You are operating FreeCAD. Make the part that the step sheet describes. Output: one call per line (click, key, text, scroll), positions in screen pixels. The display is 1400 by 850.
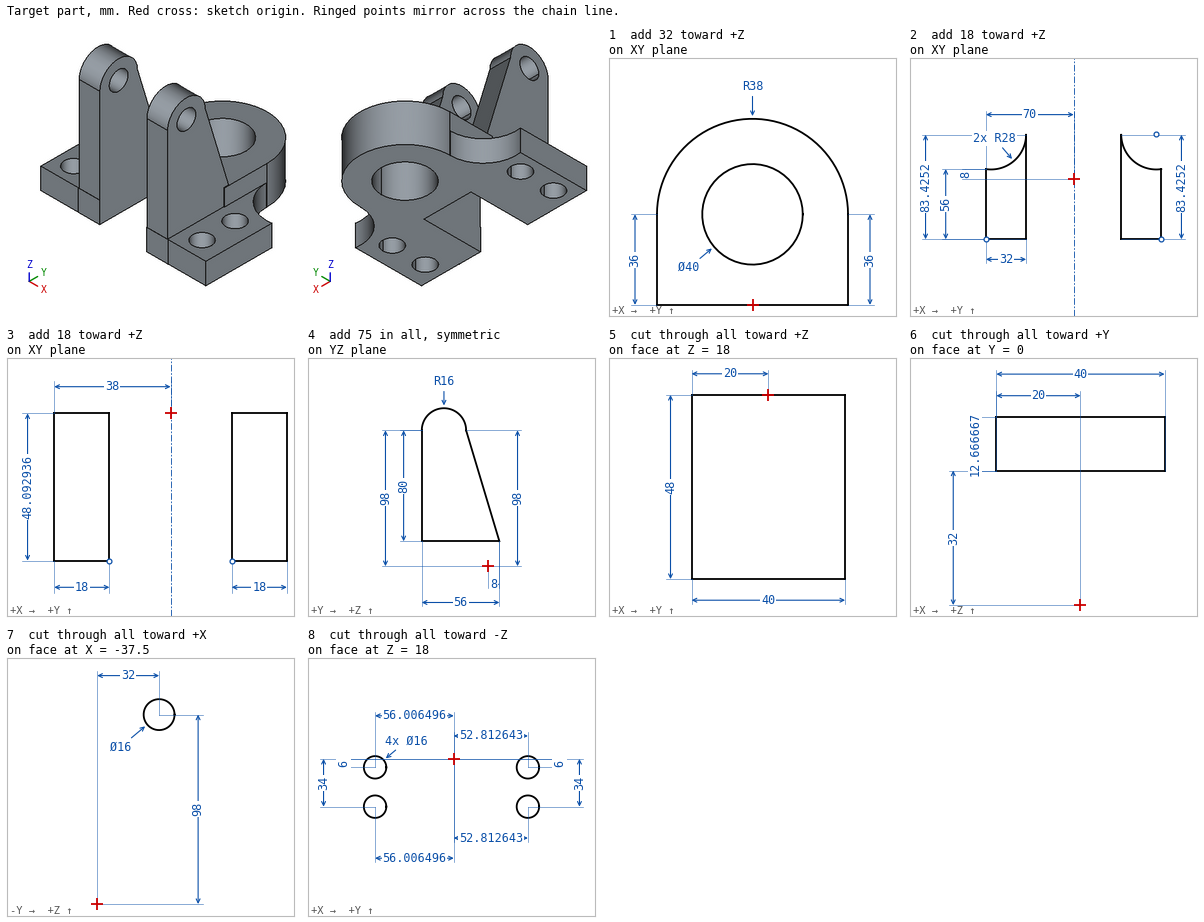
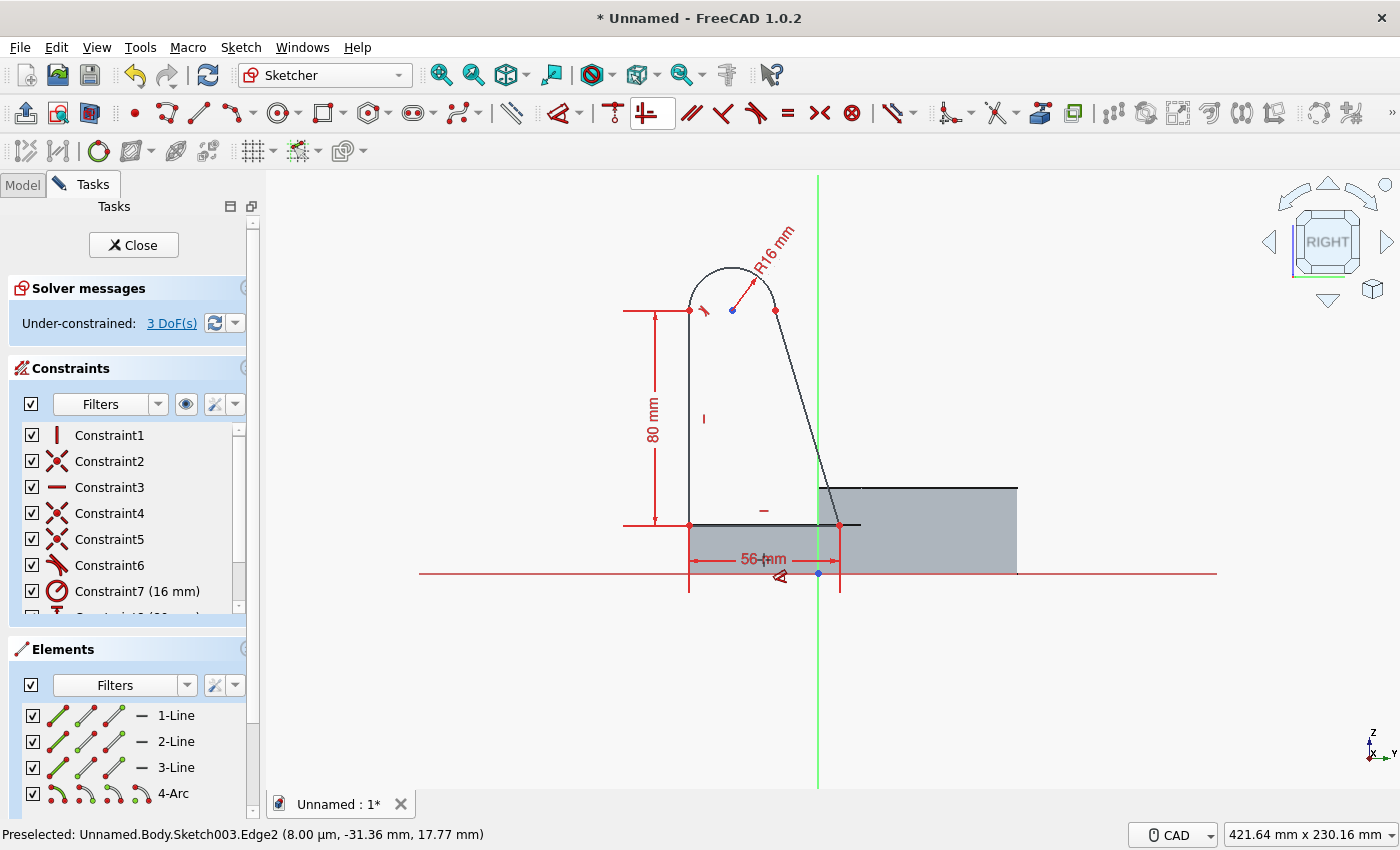
scroll(840, 526, up, 4)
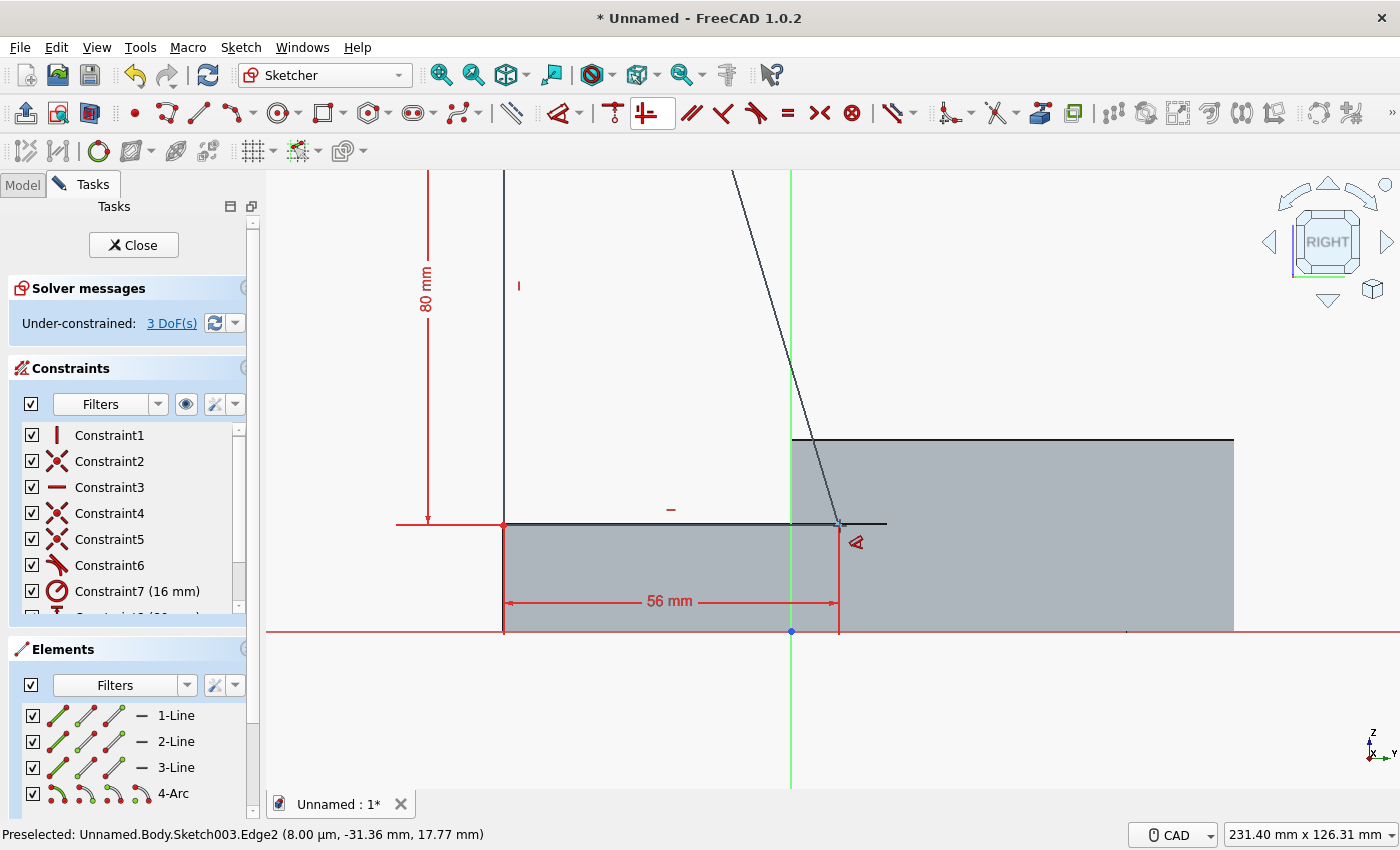
click(839, 525)
click(815, 666)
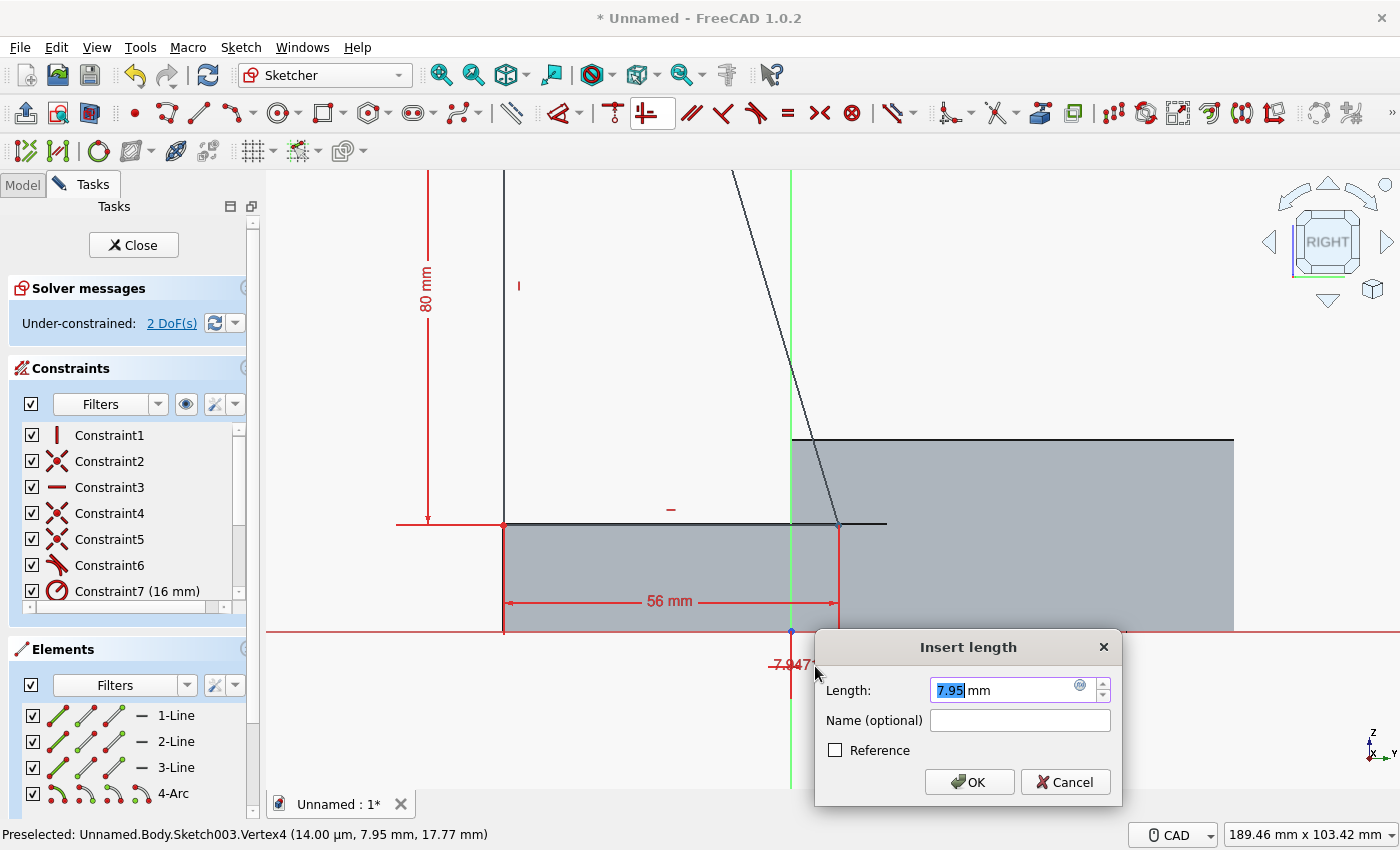
text(8)
key(Return)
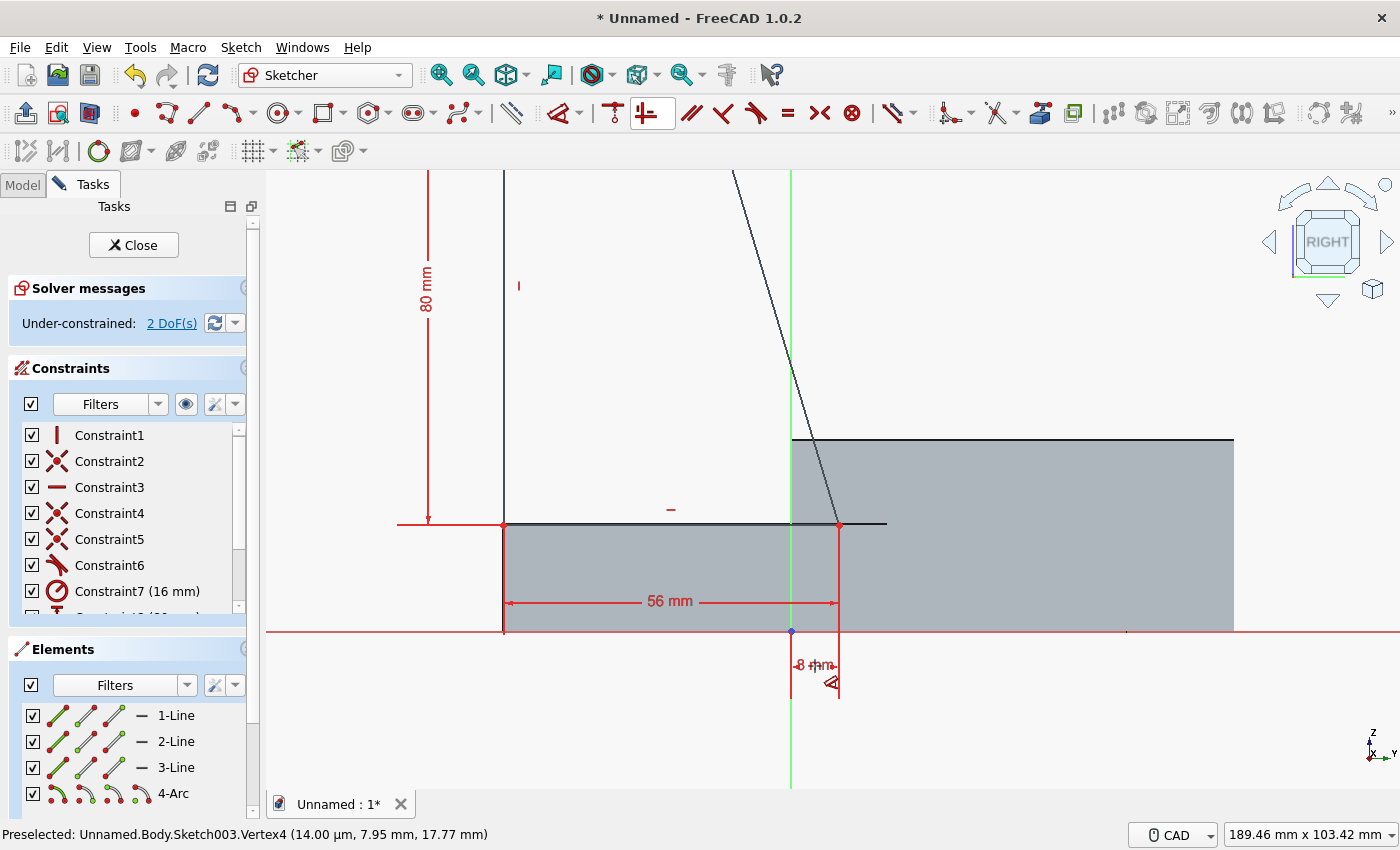
scroll(878, 709, down, 3)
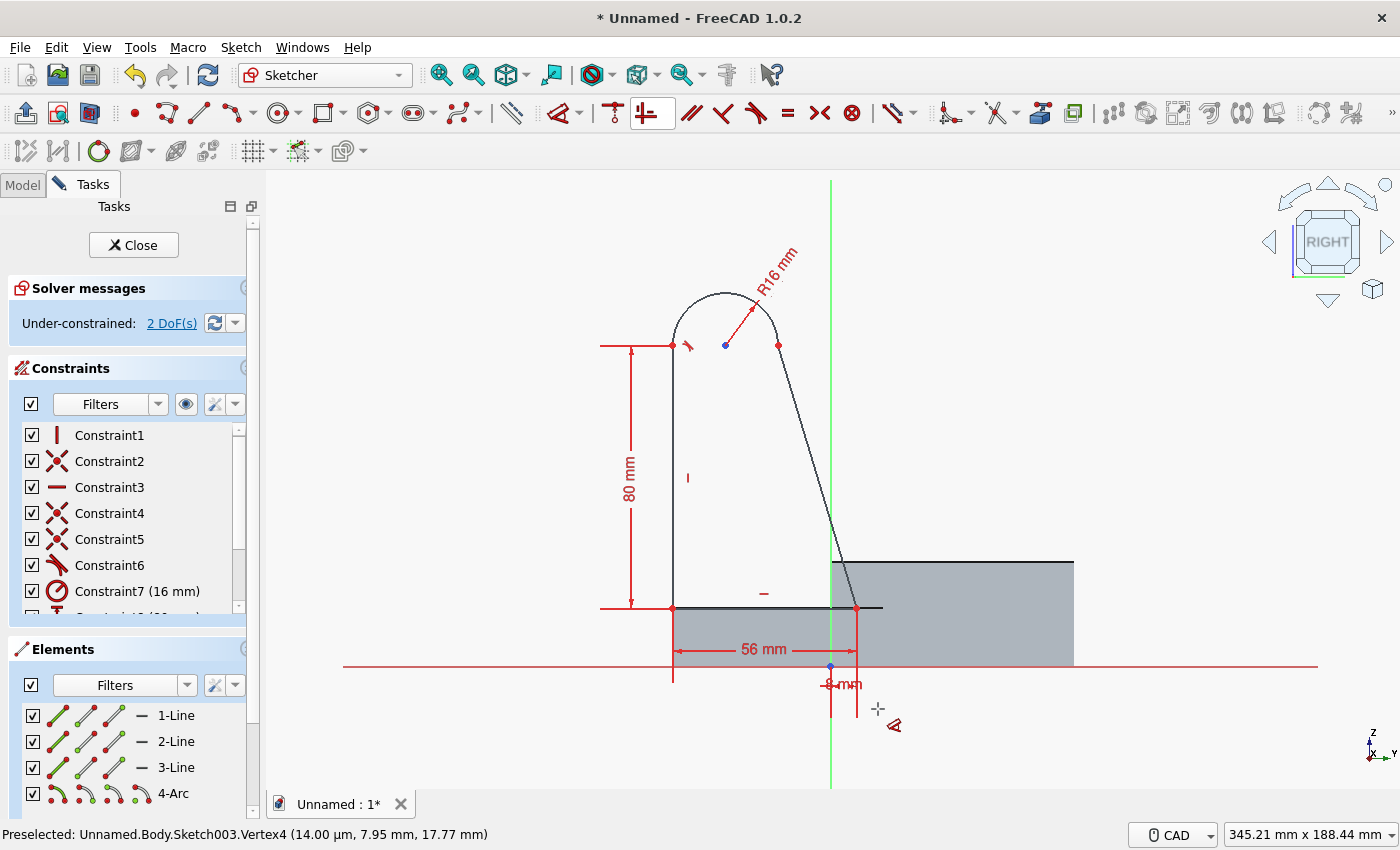
click(673, 346)
click(639, 506)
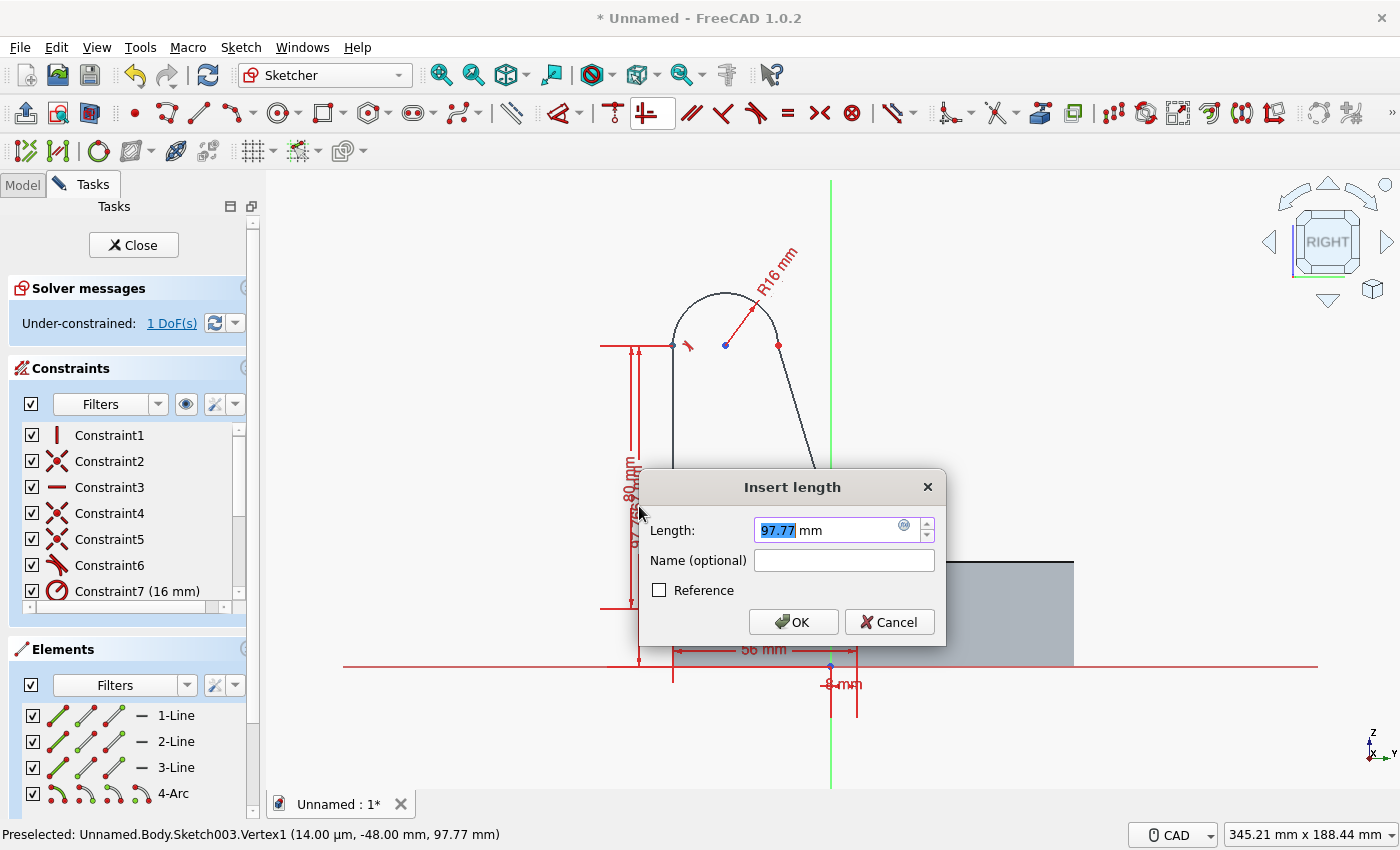
text(98)
key(Return)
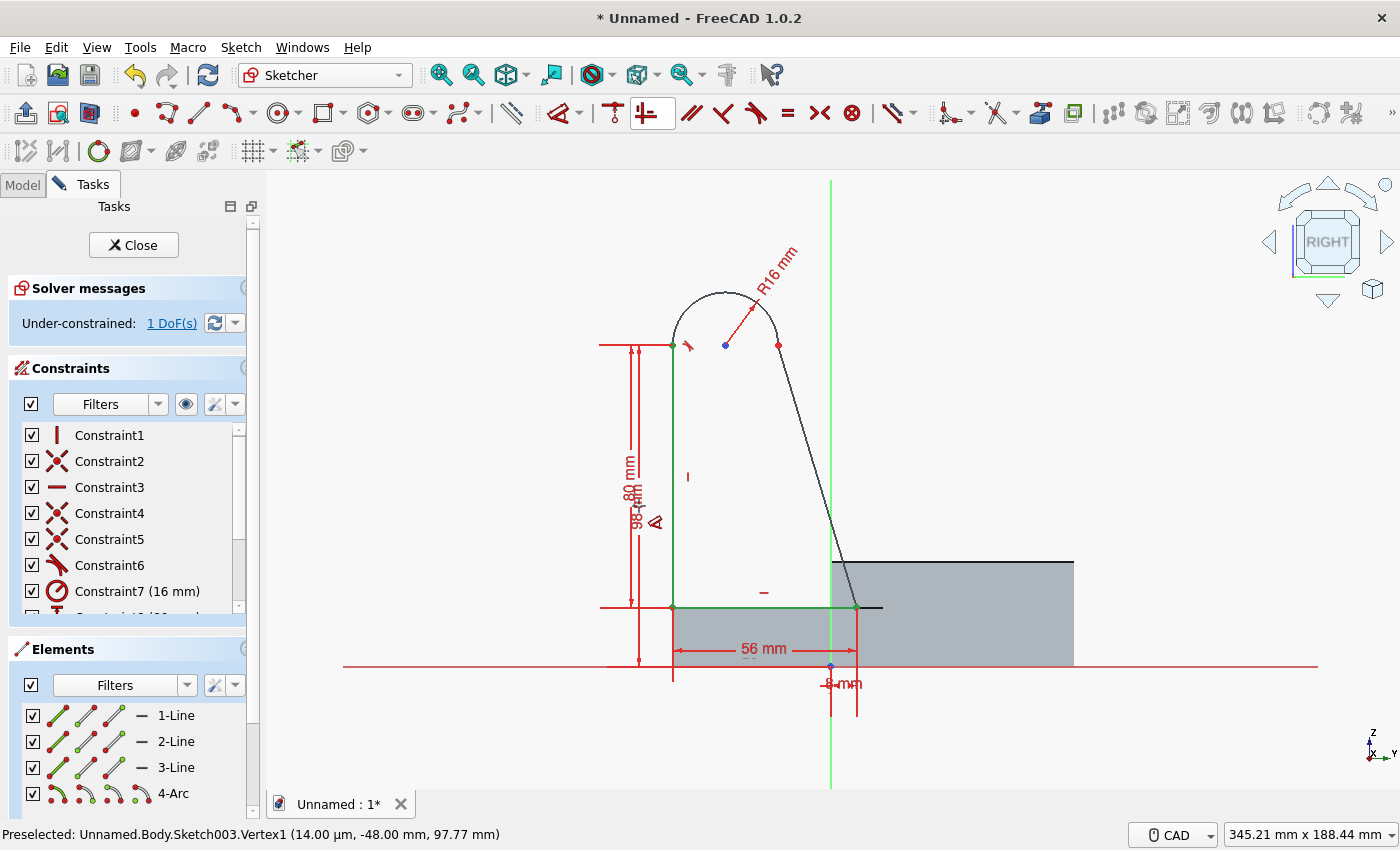
click(778, 346)
click(865, 506)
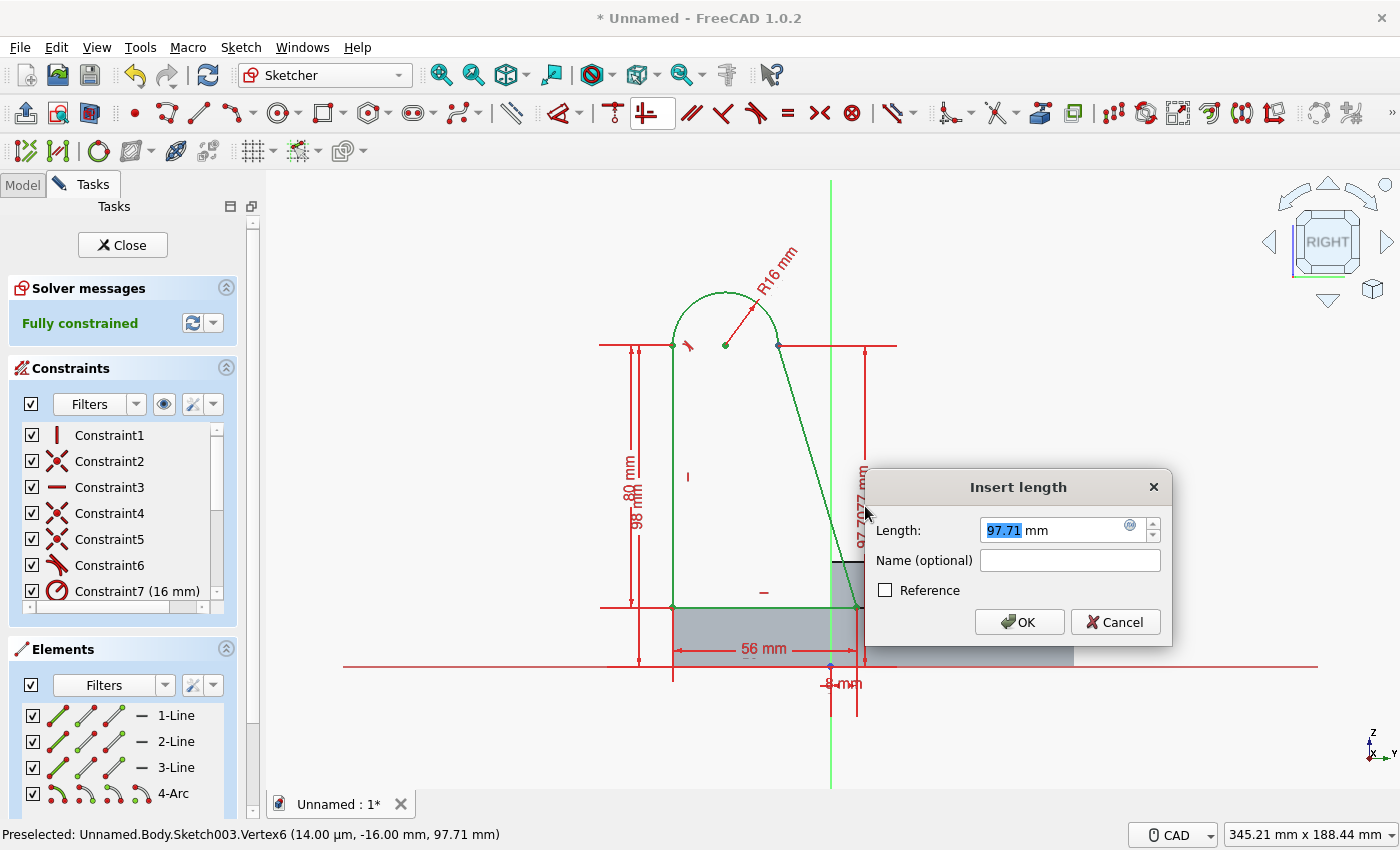
text(98)
key(Return)
key(Escape)